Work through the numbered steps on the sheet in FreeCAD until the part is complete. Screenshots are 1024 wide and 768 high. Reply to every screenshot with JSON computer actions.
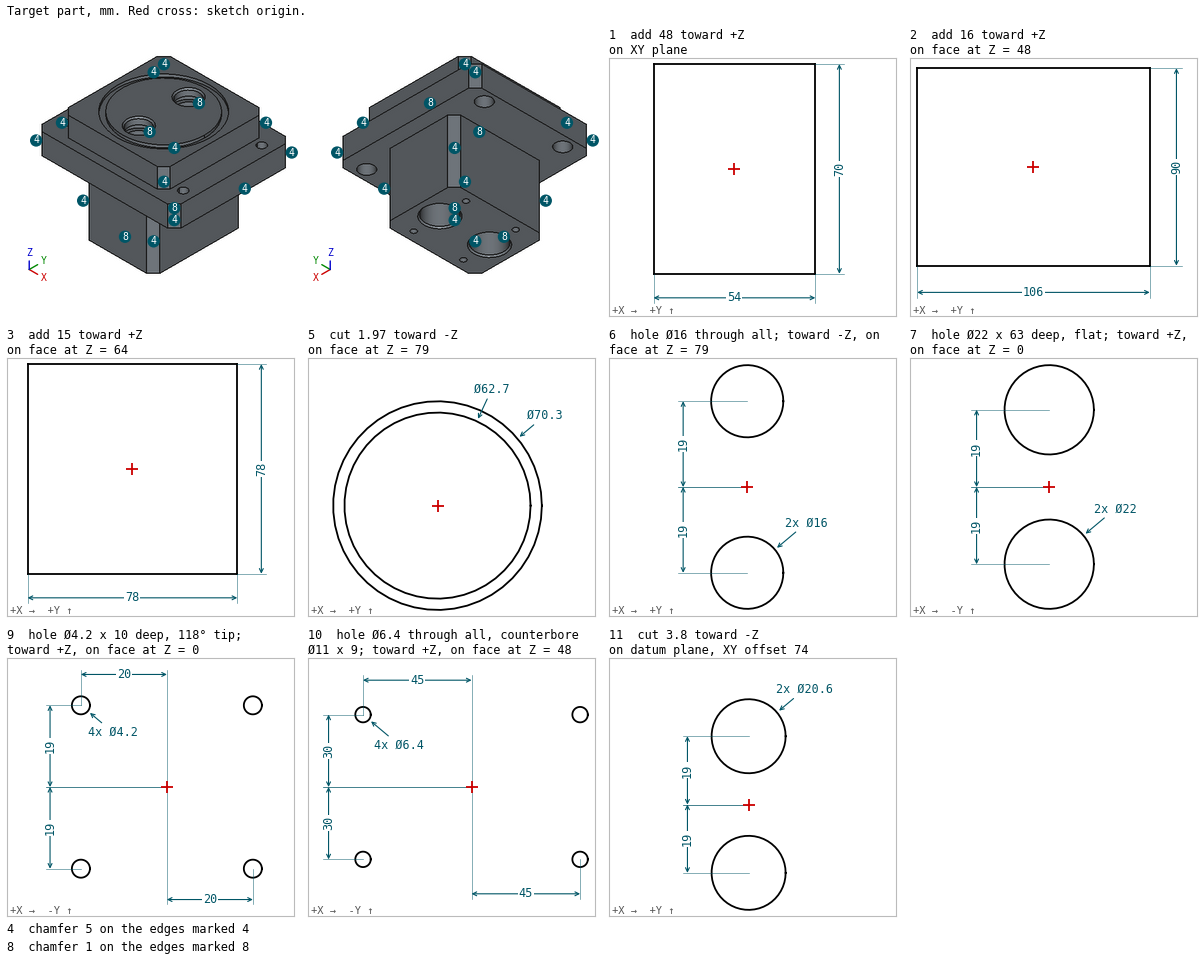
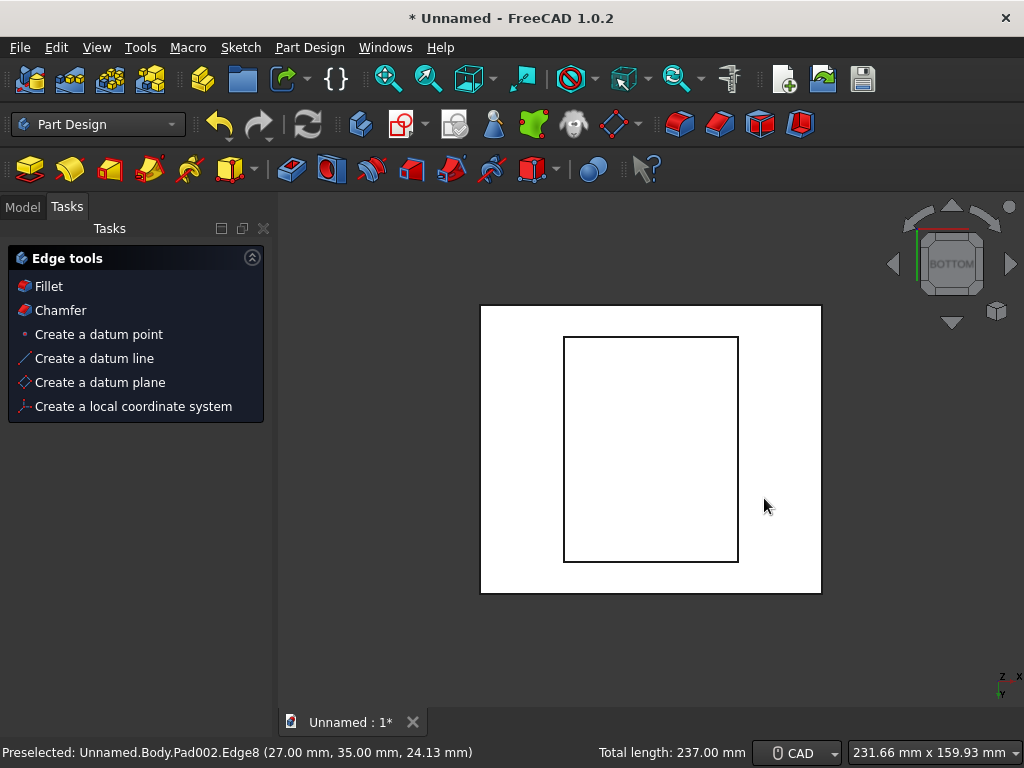
{"action": "key", "text": "4"}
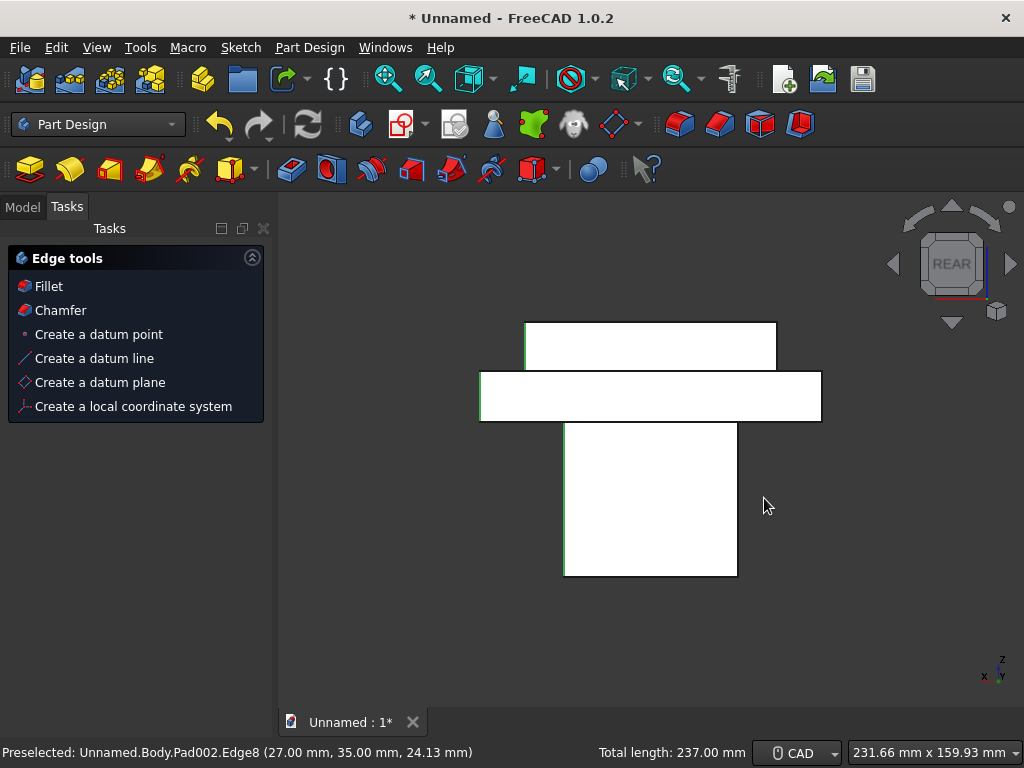
{"action": "left_click", "coordinate": [822, 395], "text": "ctrl"}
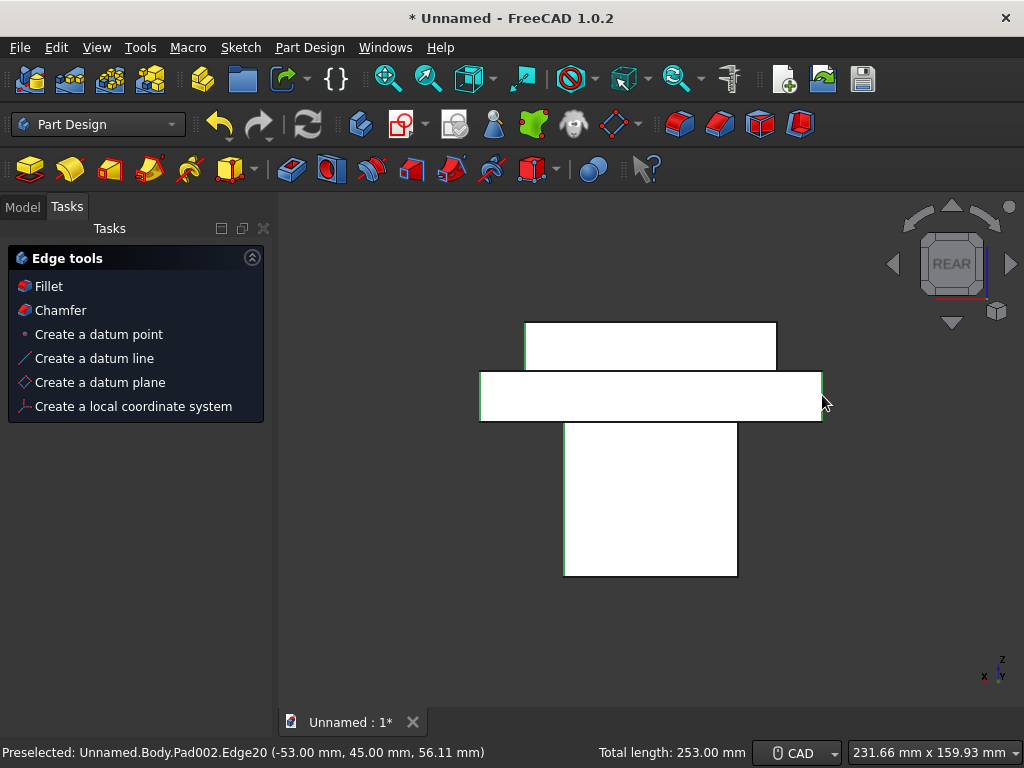
{"action": "left_click", "coordinate": [777, 345], "text": "ctrl"}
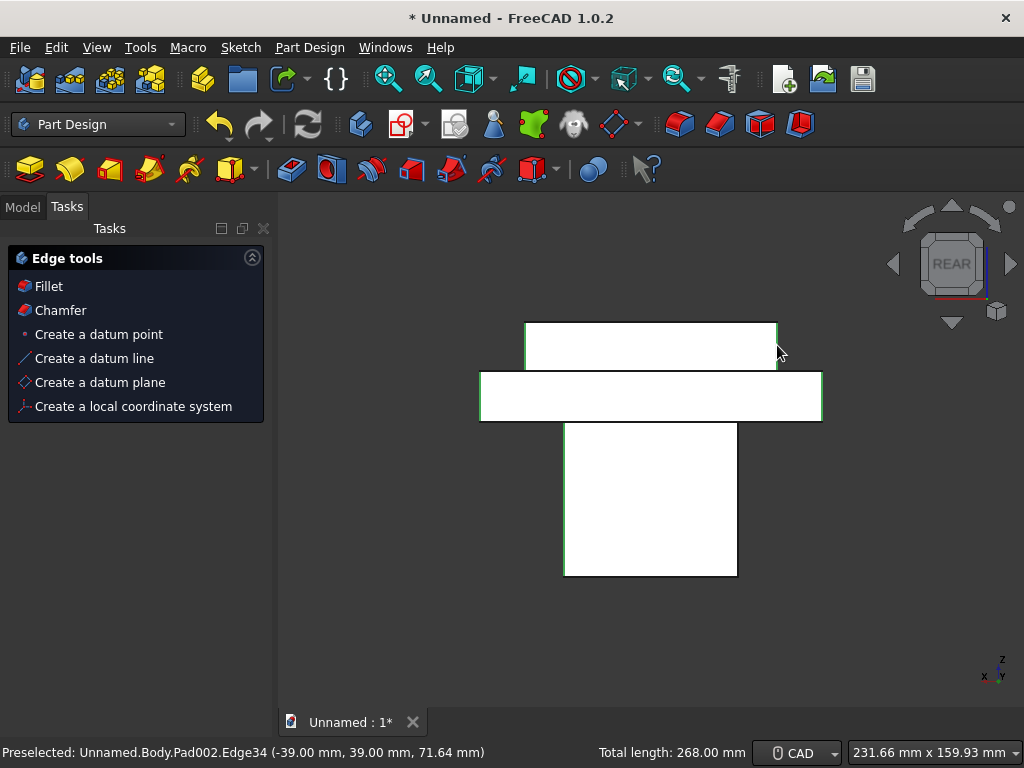
{"action": "left_click", "coordinate": [738, 498], "text": "ctrl"}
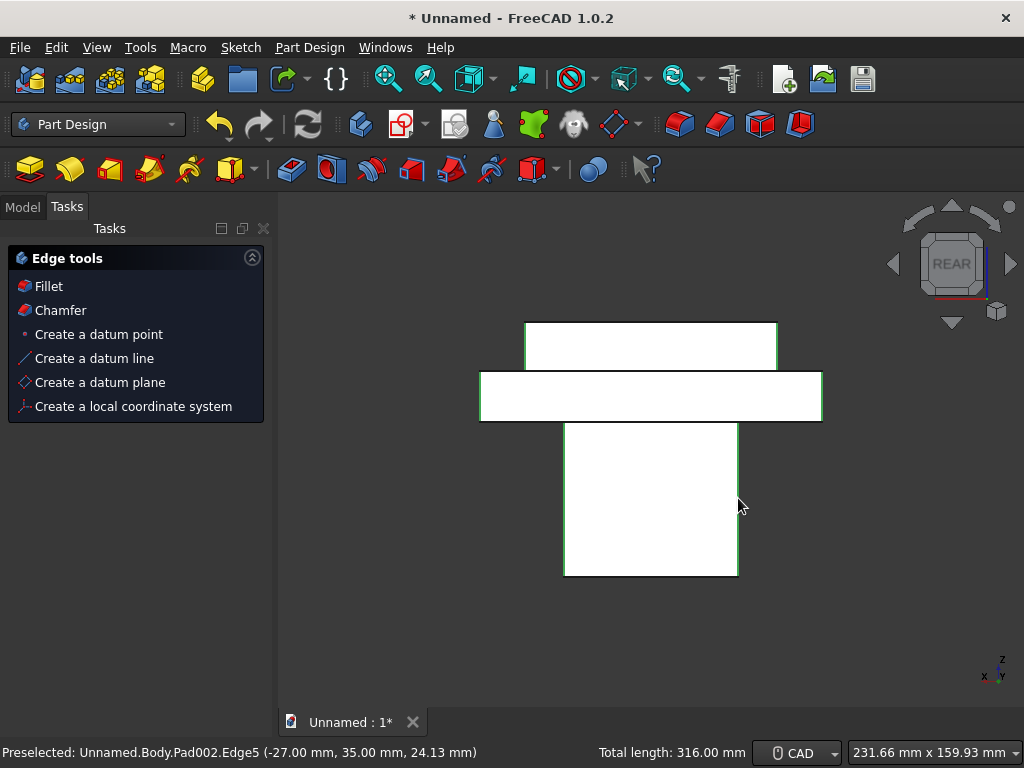
{"action": "left_click", "coordinate": [720, 124]}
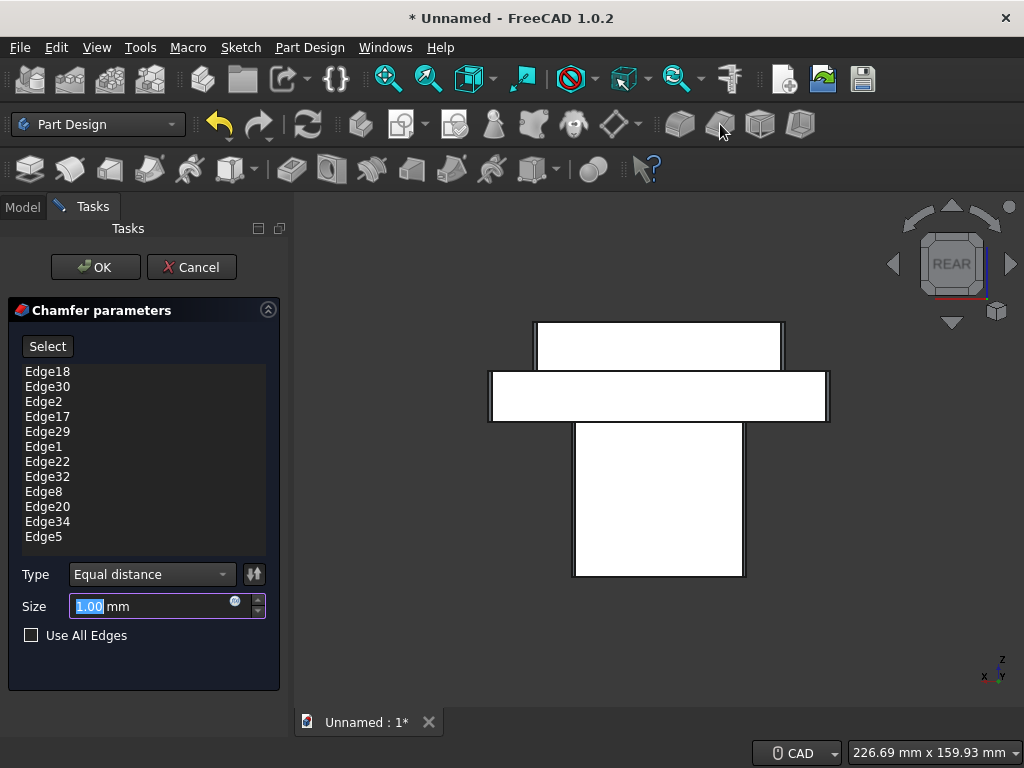
{"action": "type", "text": "5"}
{"action": "key", "text": "Tab"}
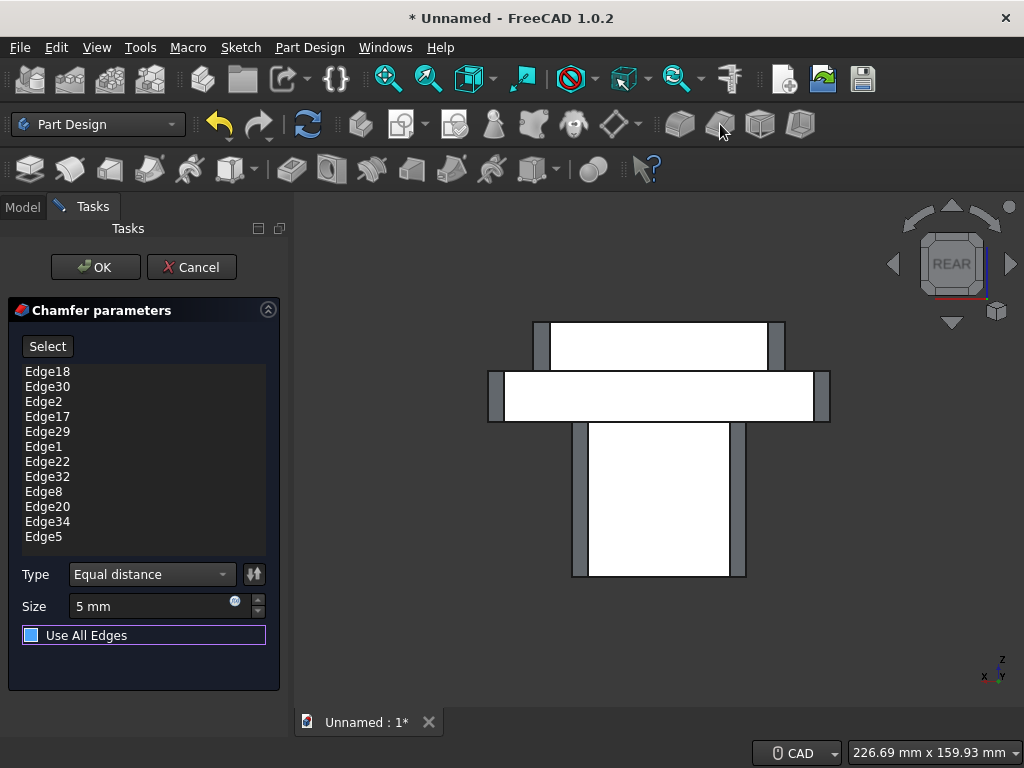
{"action": "left_click", "coordinate": [96, 267]}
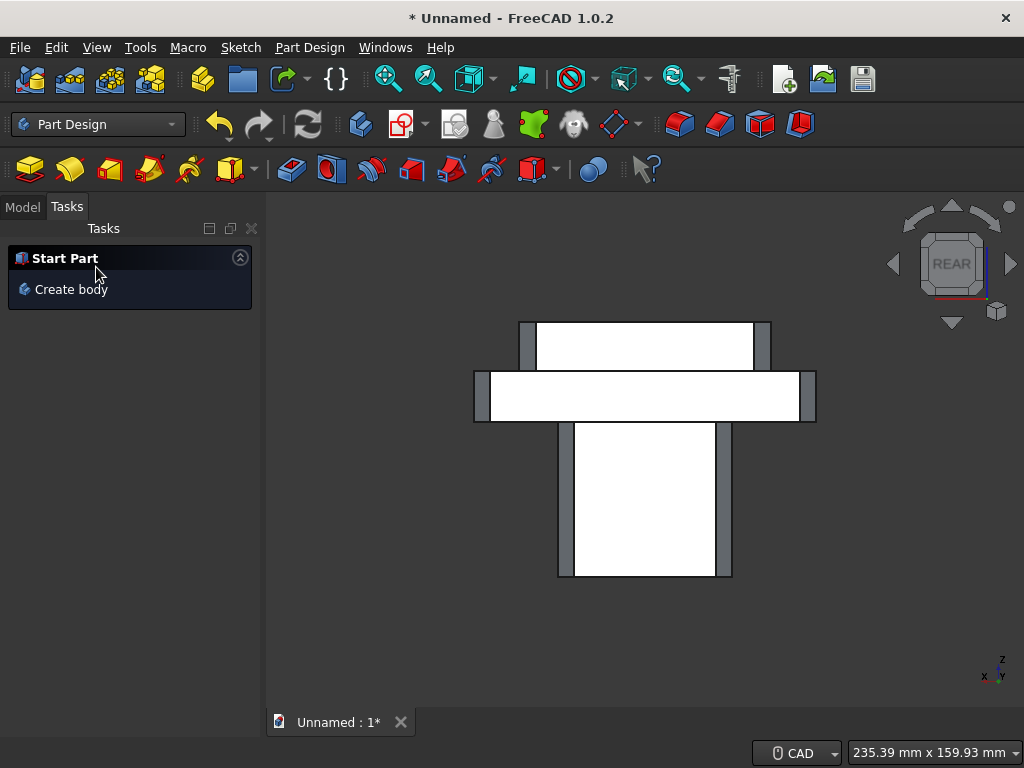
{"action": "key", "text": "0"}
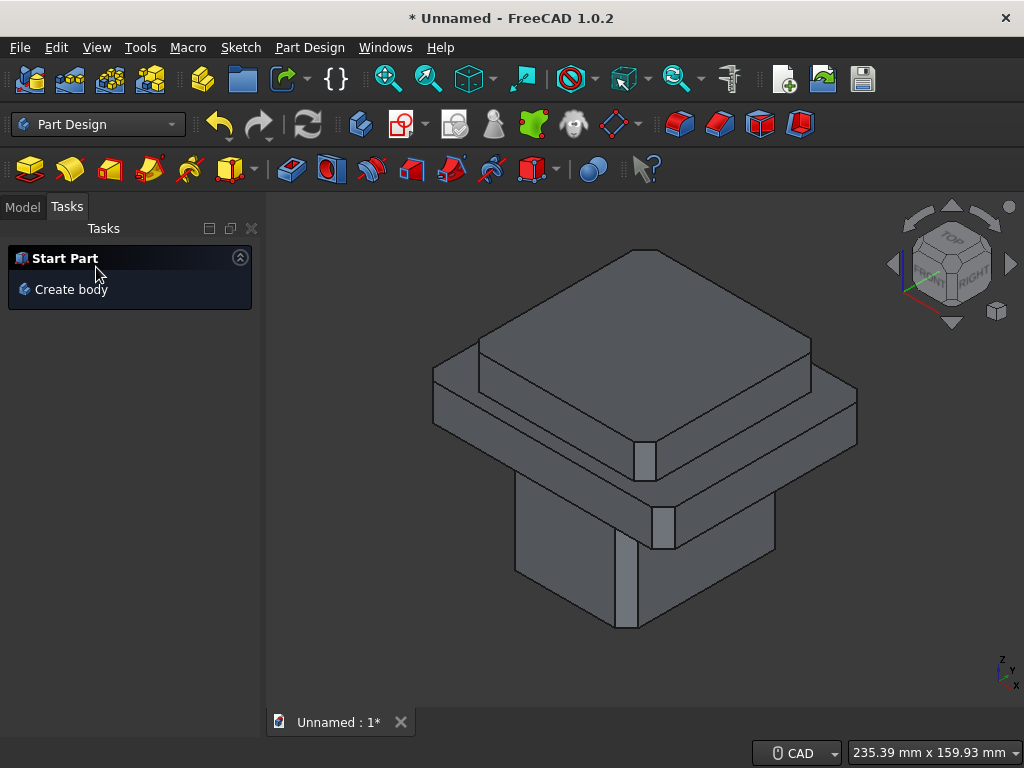
{"action": "left_click", "coordinate": [645, 345]}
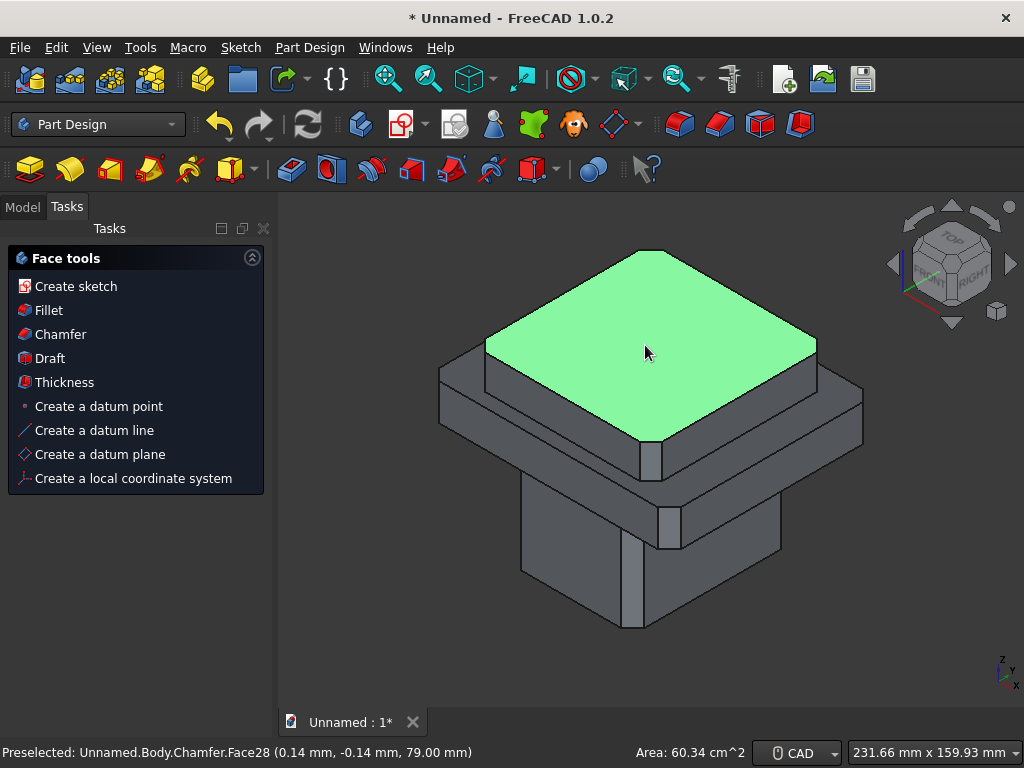
{"action": "left_click", "coordinate": [402, 124]}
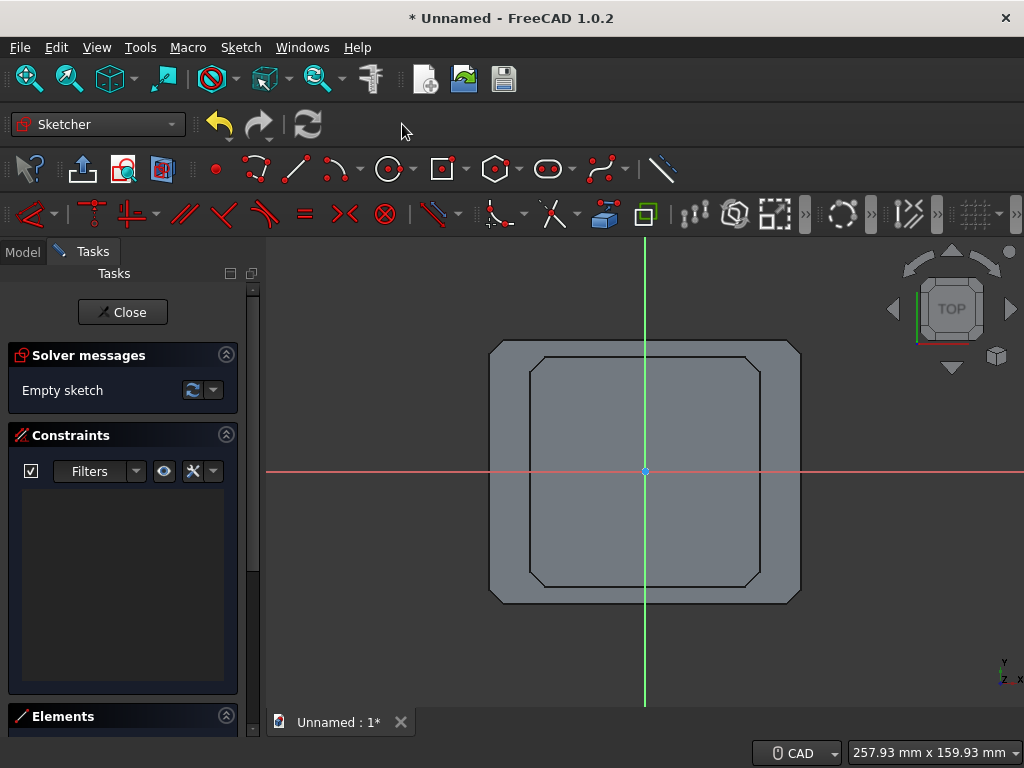
{"action": "scroll", "coordinate": [784, 472], "scroll_direction": "up", "scroll_amount": 2}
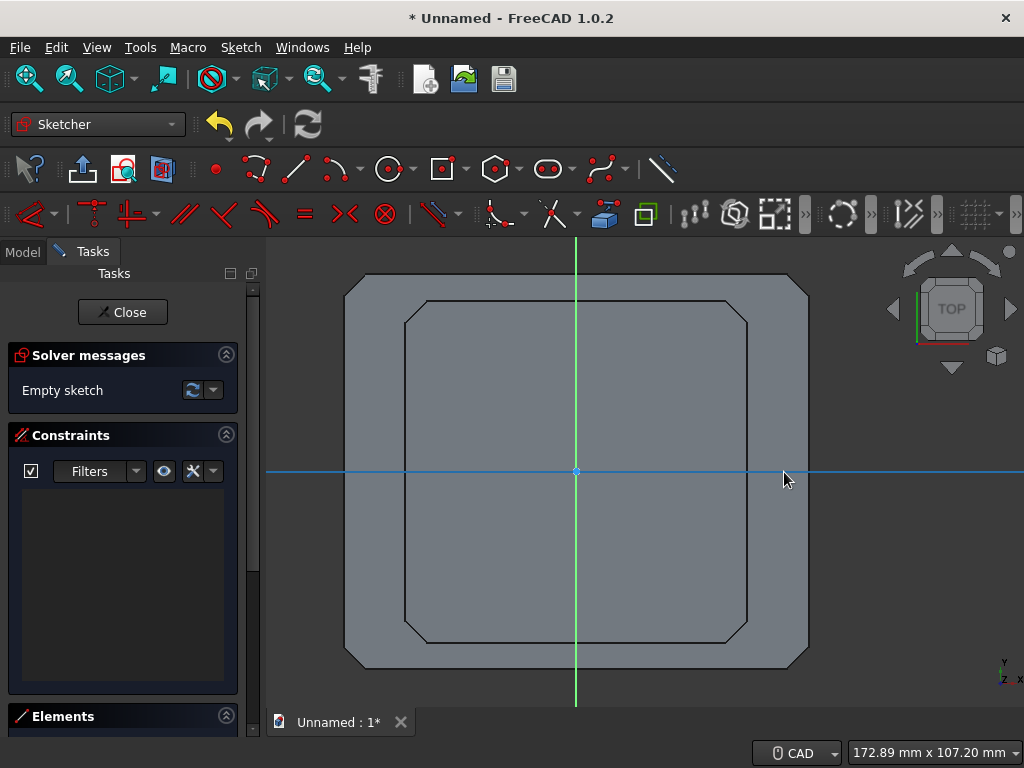
{"action": "left_click", "coordinate": [390, 170]}